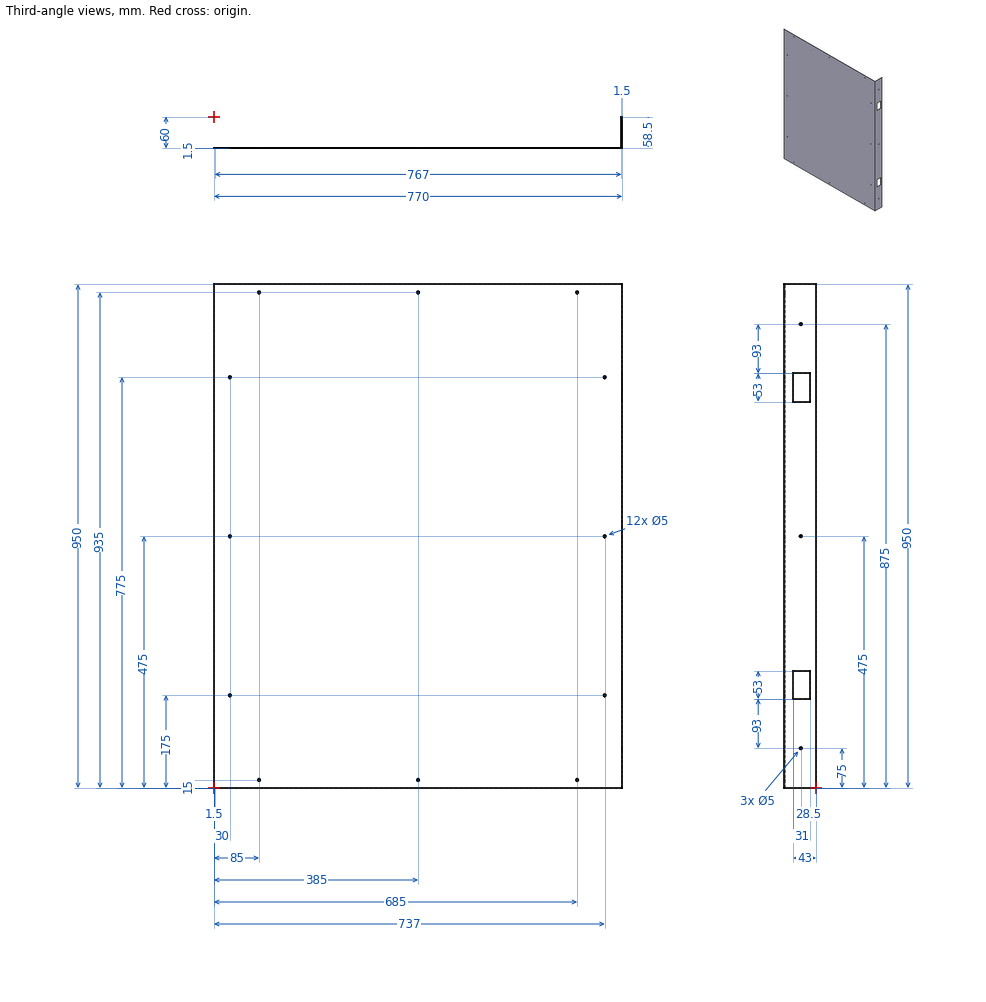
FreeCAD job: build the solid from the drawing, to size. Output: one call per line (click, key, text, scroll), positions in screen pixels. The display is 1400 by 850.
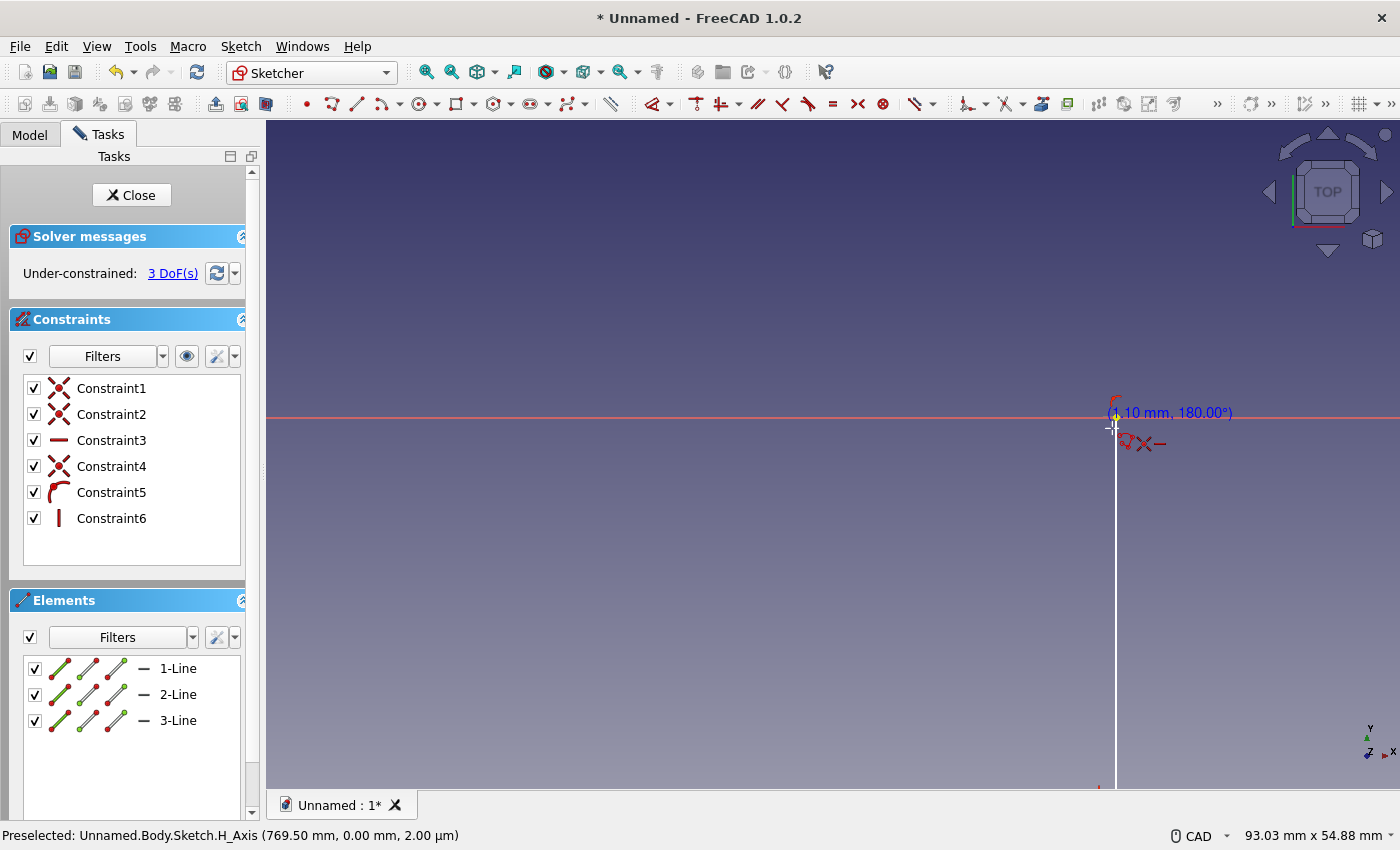
click(1104, 427)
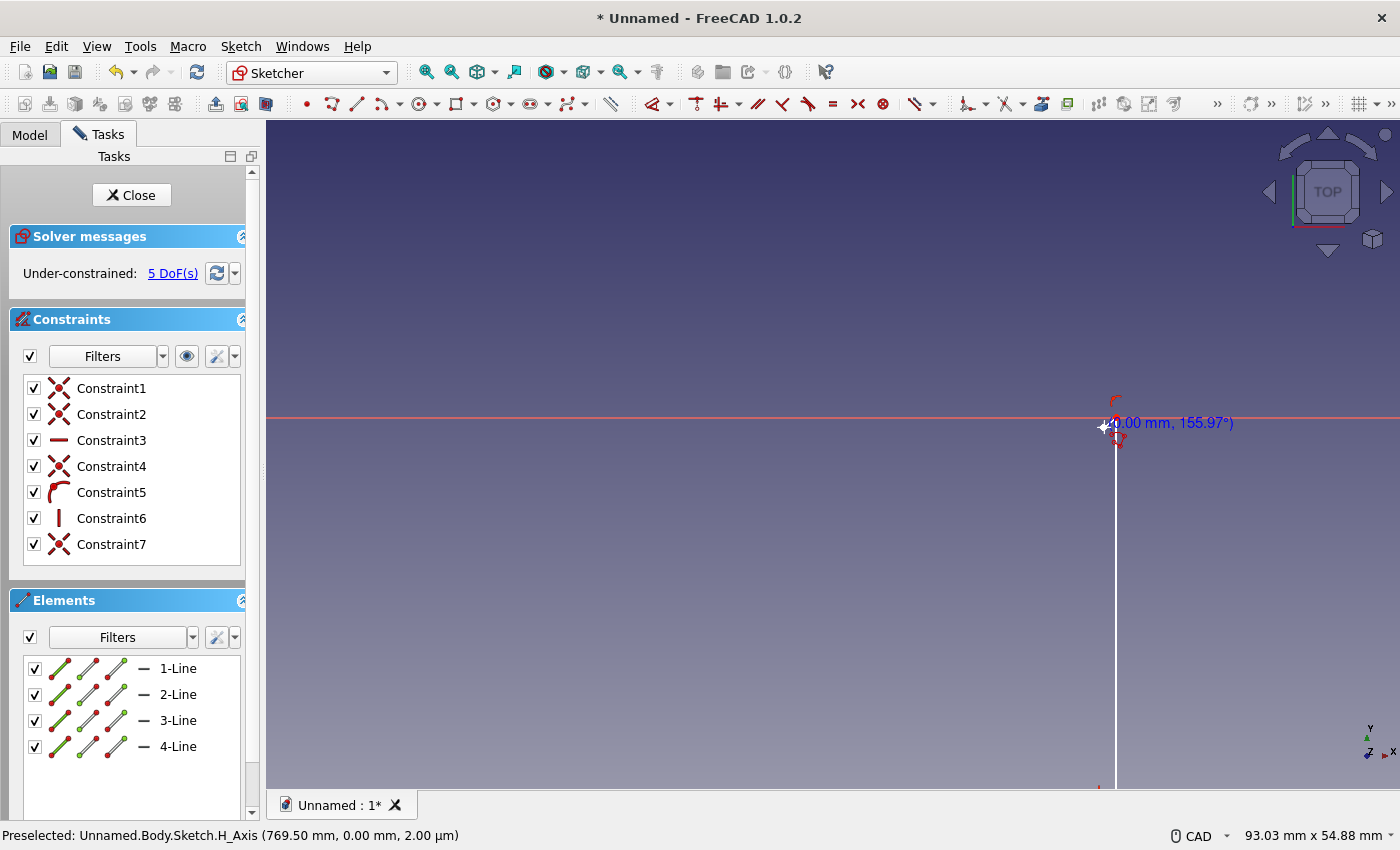
scroll(1112, 428, down, 13)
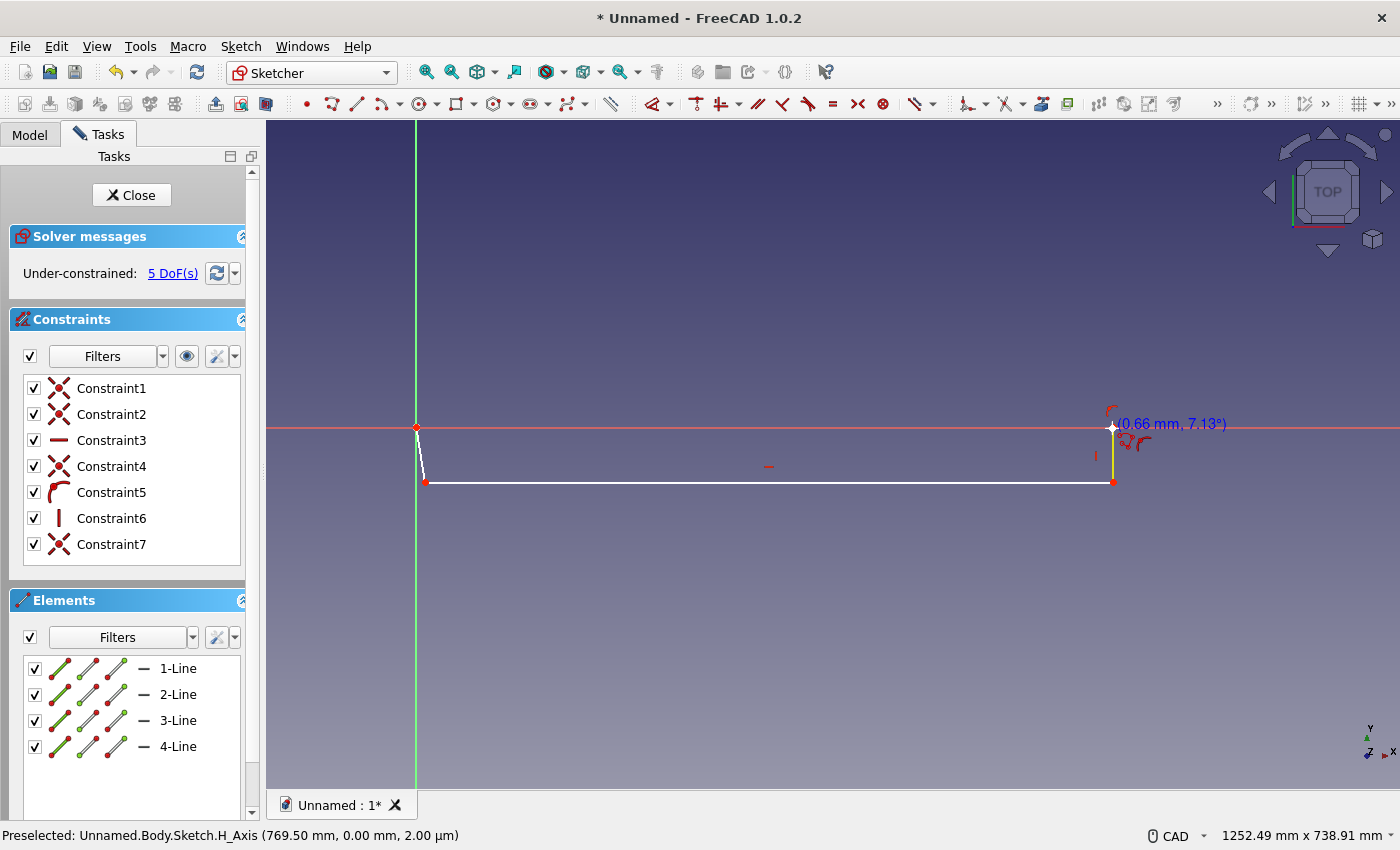
scroll(1112, 481, up, 13)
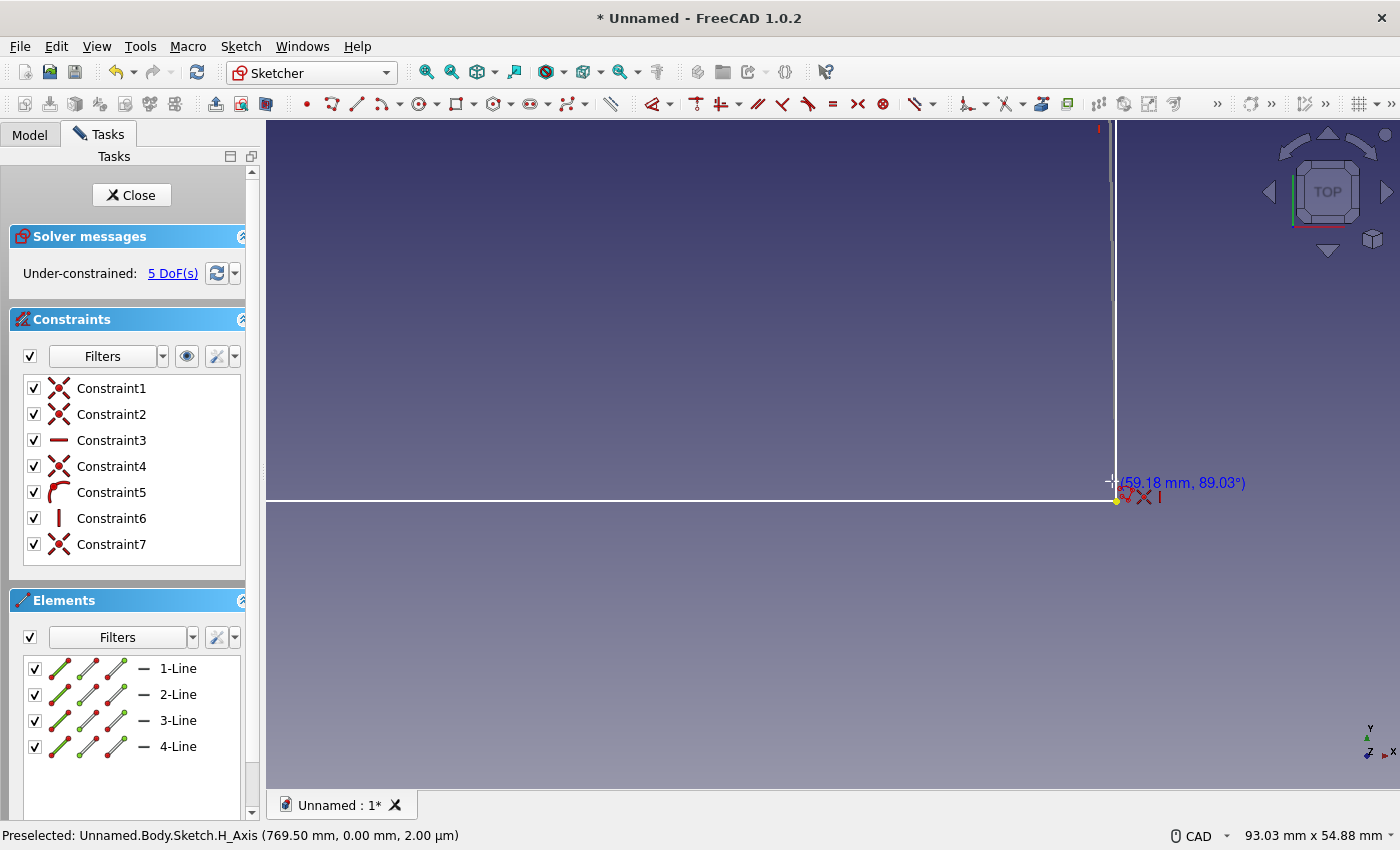
click(1104, 469)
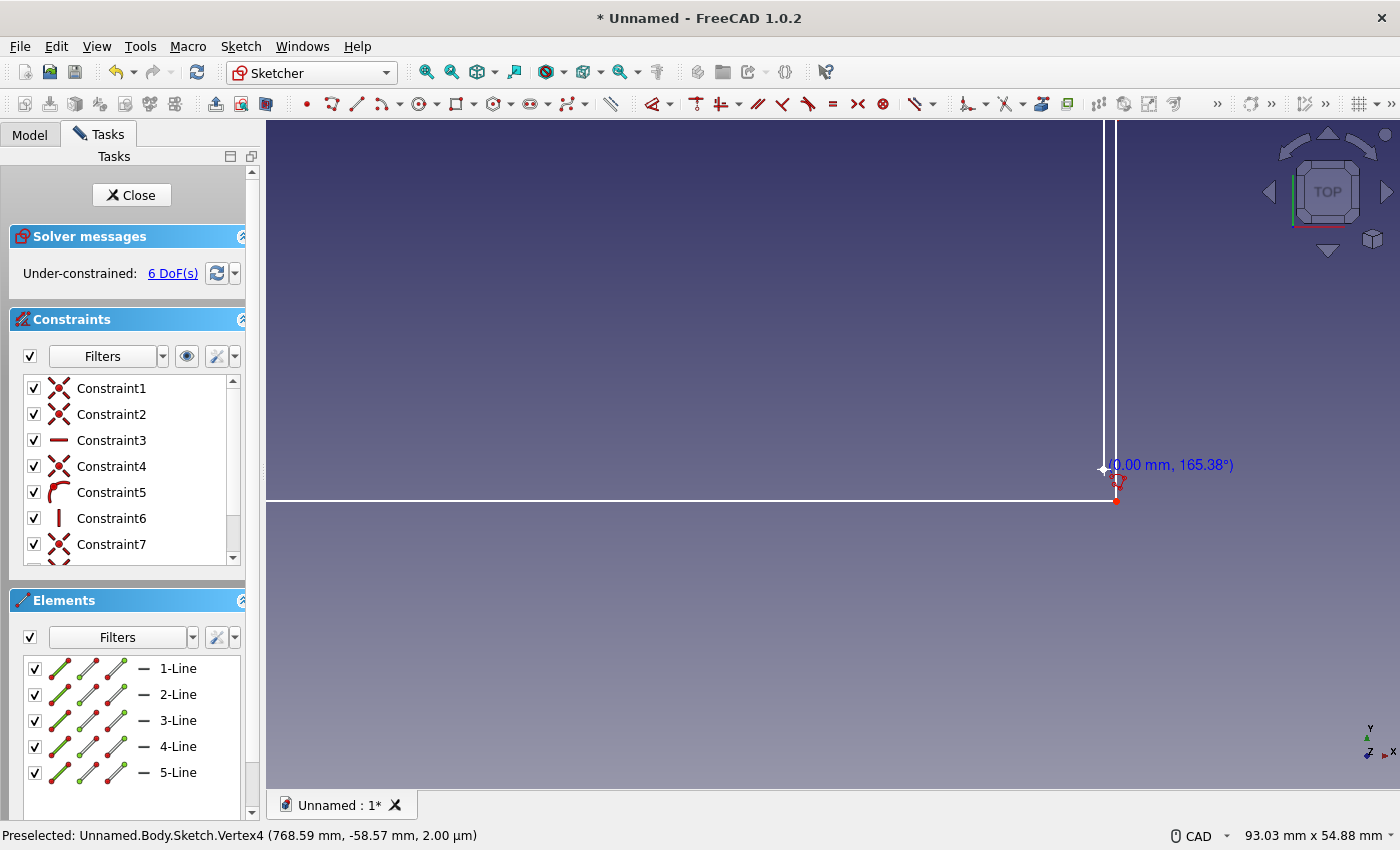
scroll(1112, 481, down, 13)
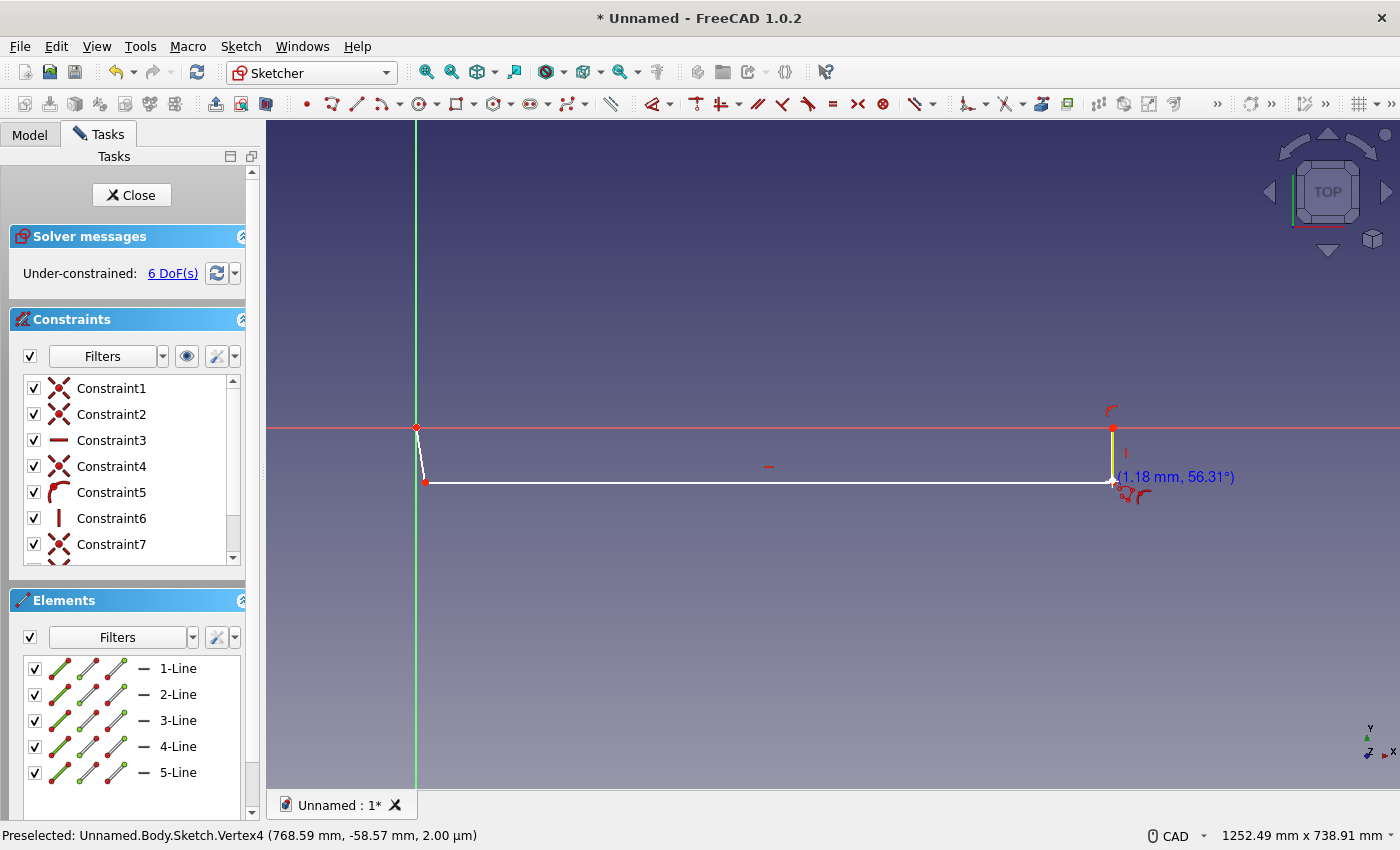
scroll(418, 481, up, 13)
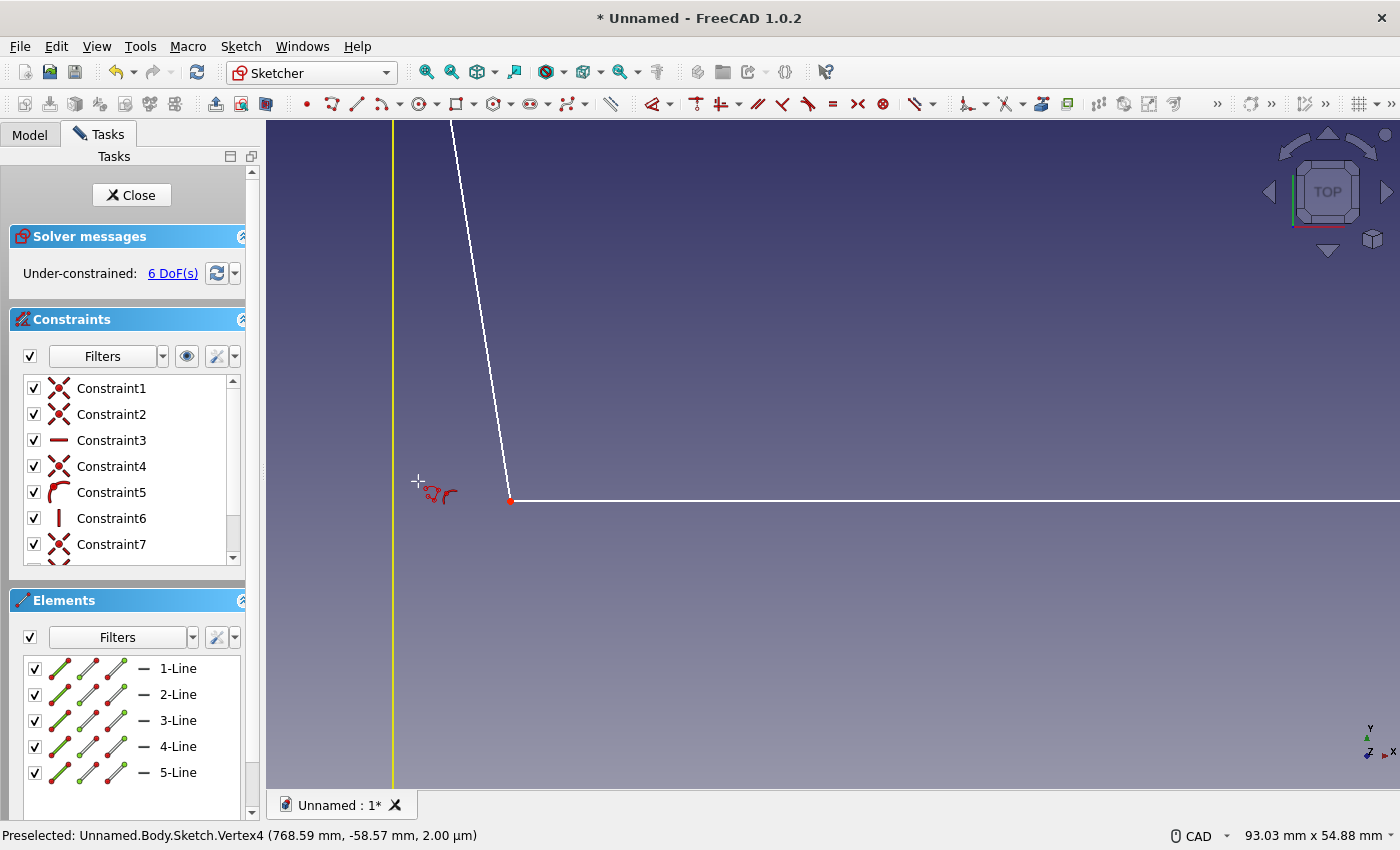
click(412, 469)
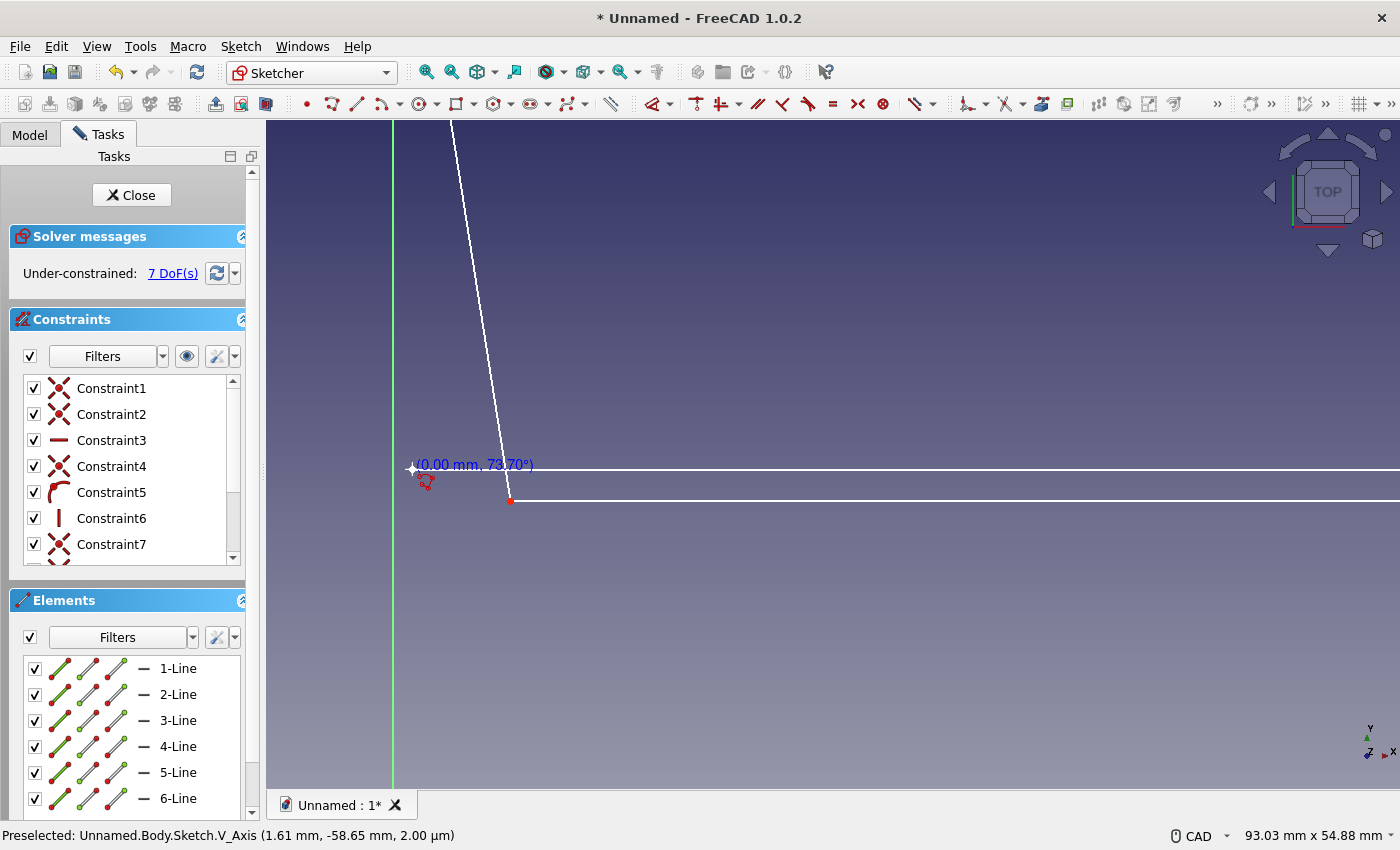
scroll(418, 481, down, 13)